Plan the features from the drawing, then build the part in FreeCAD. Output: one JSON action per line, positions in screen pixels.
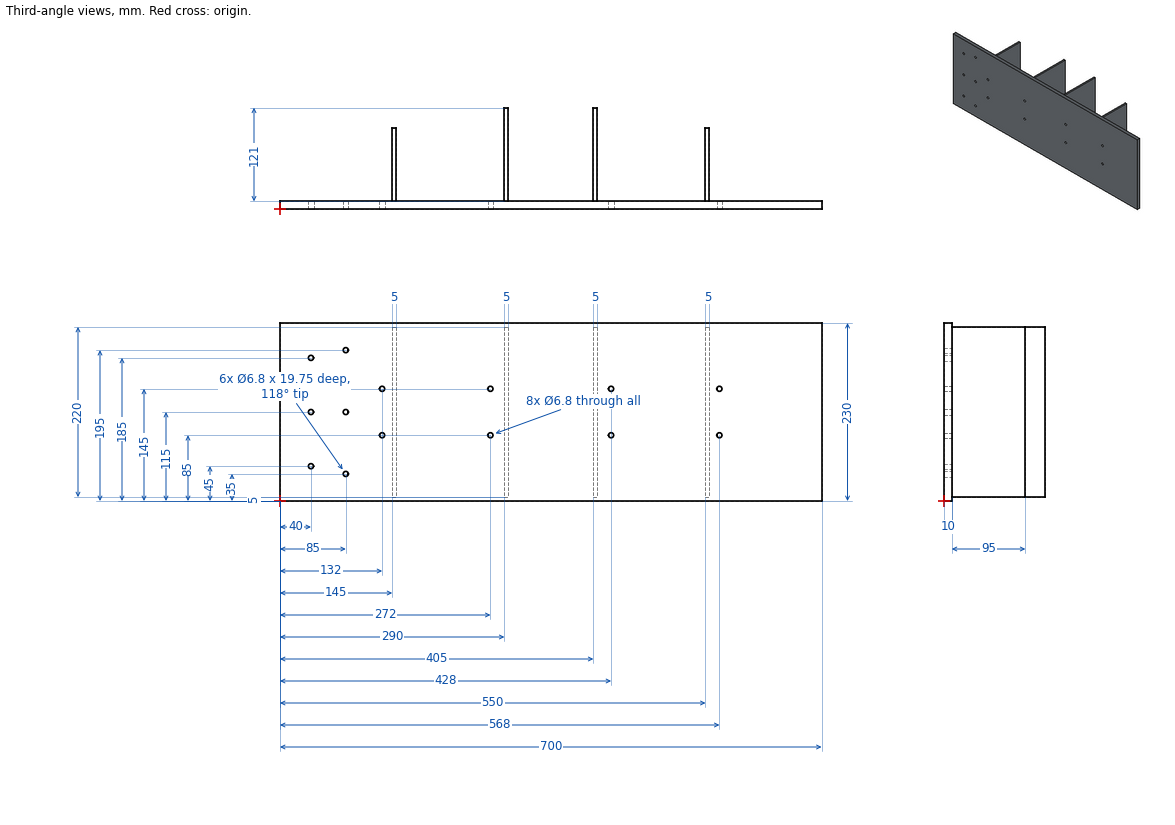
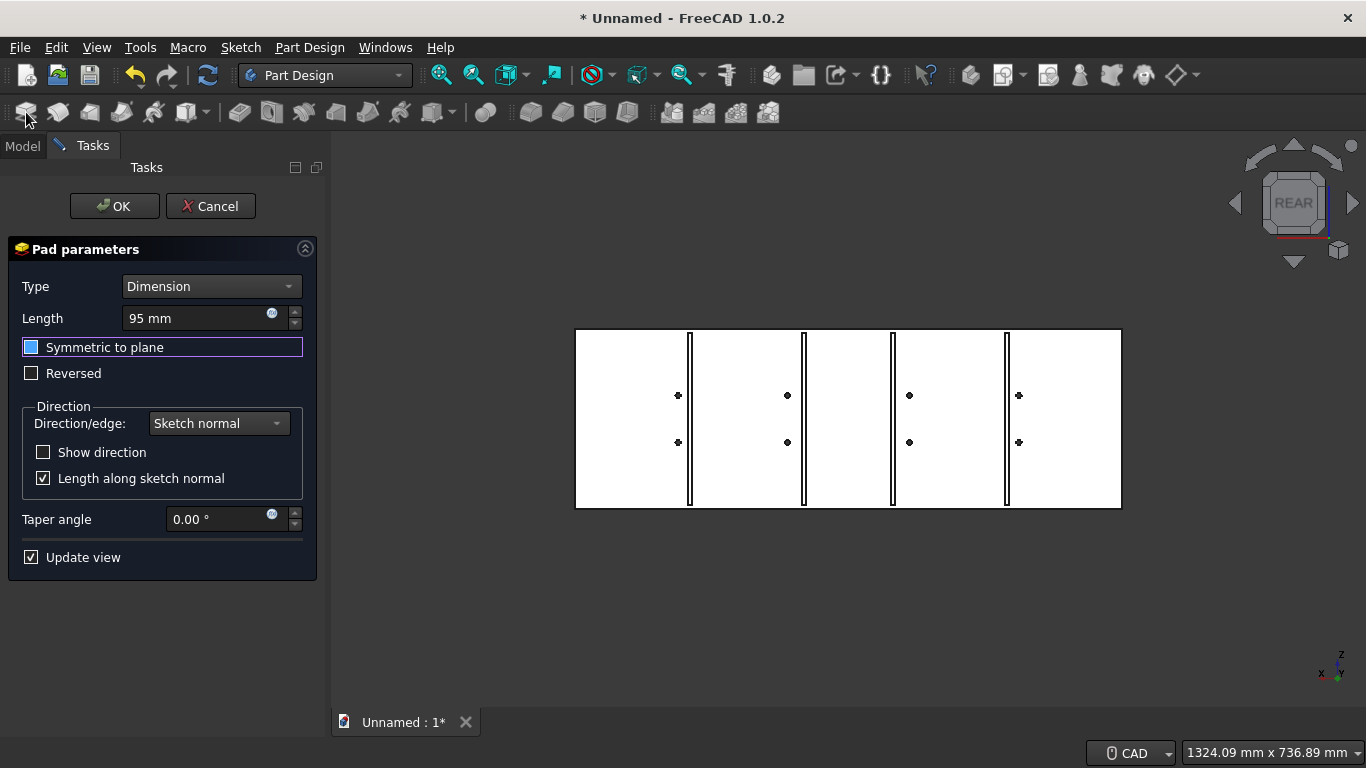
{"action": "left_click", "coordinate": [115, 206]}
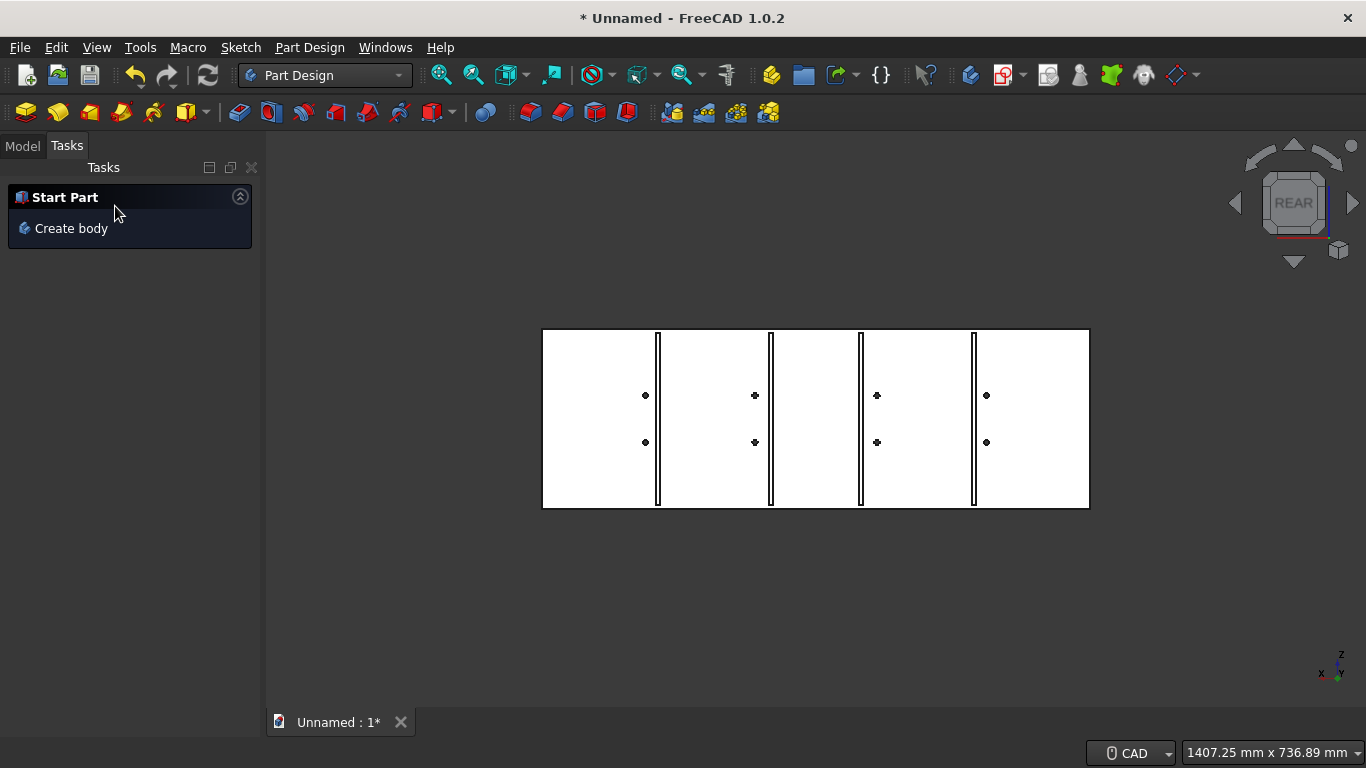
{"action": "left_click", "coordinate": [1004, 76]}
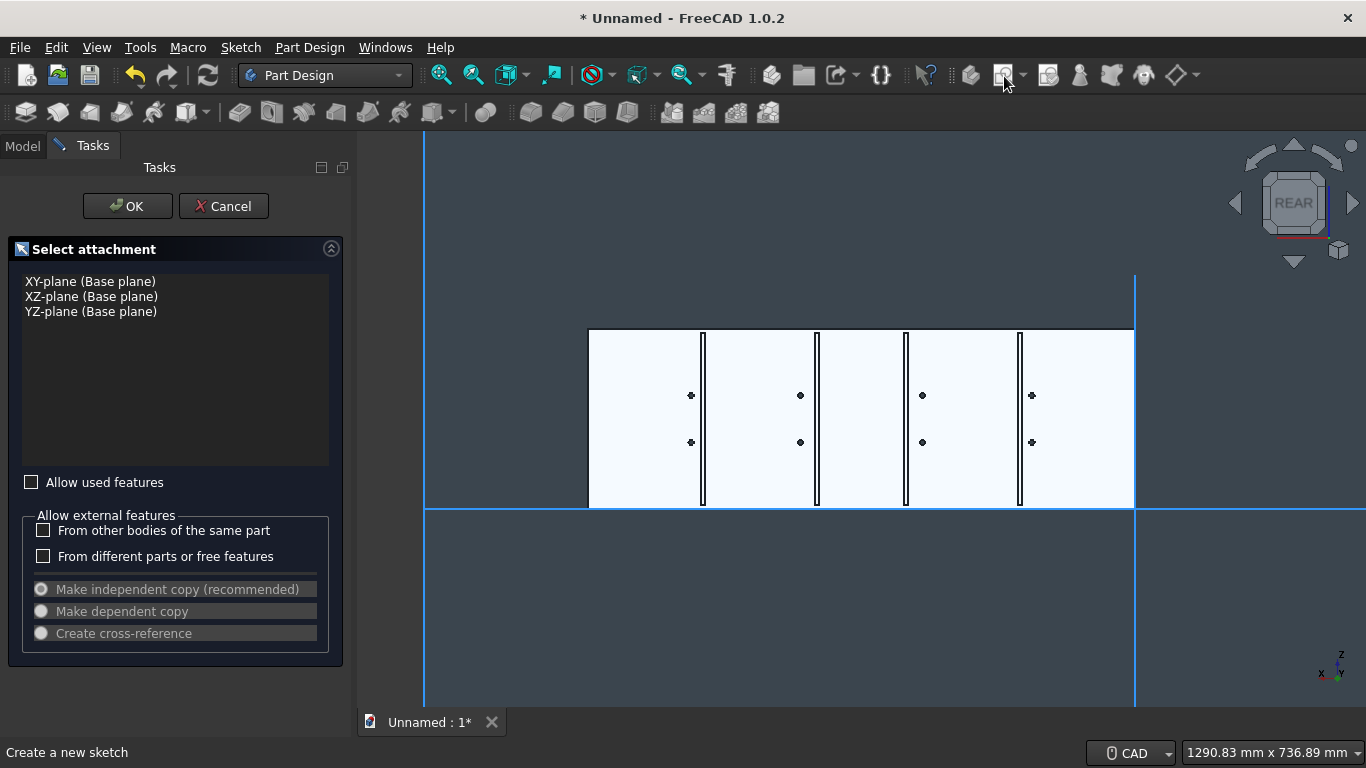
{"action": "left_click", "coordinate": [82, 296]}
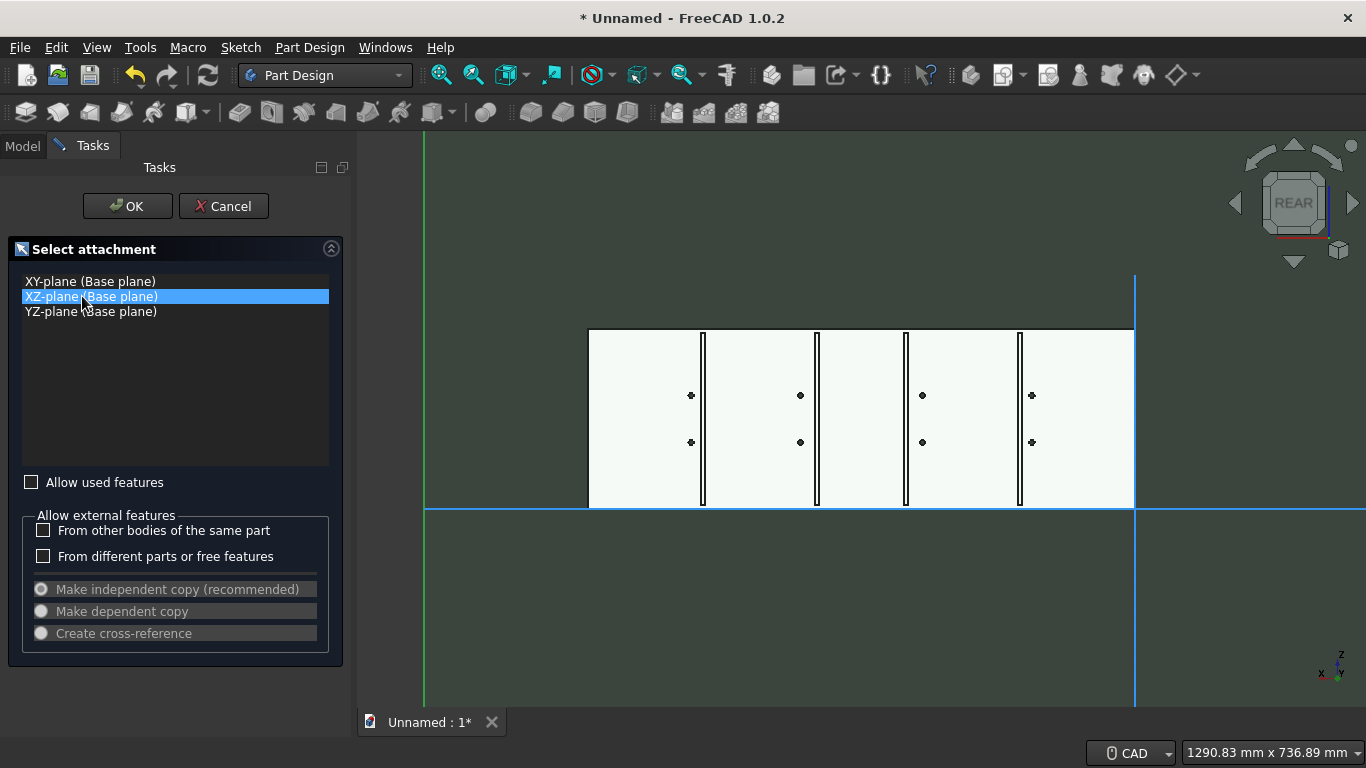
{"action": "left_click", "coordinate": [128, 206]}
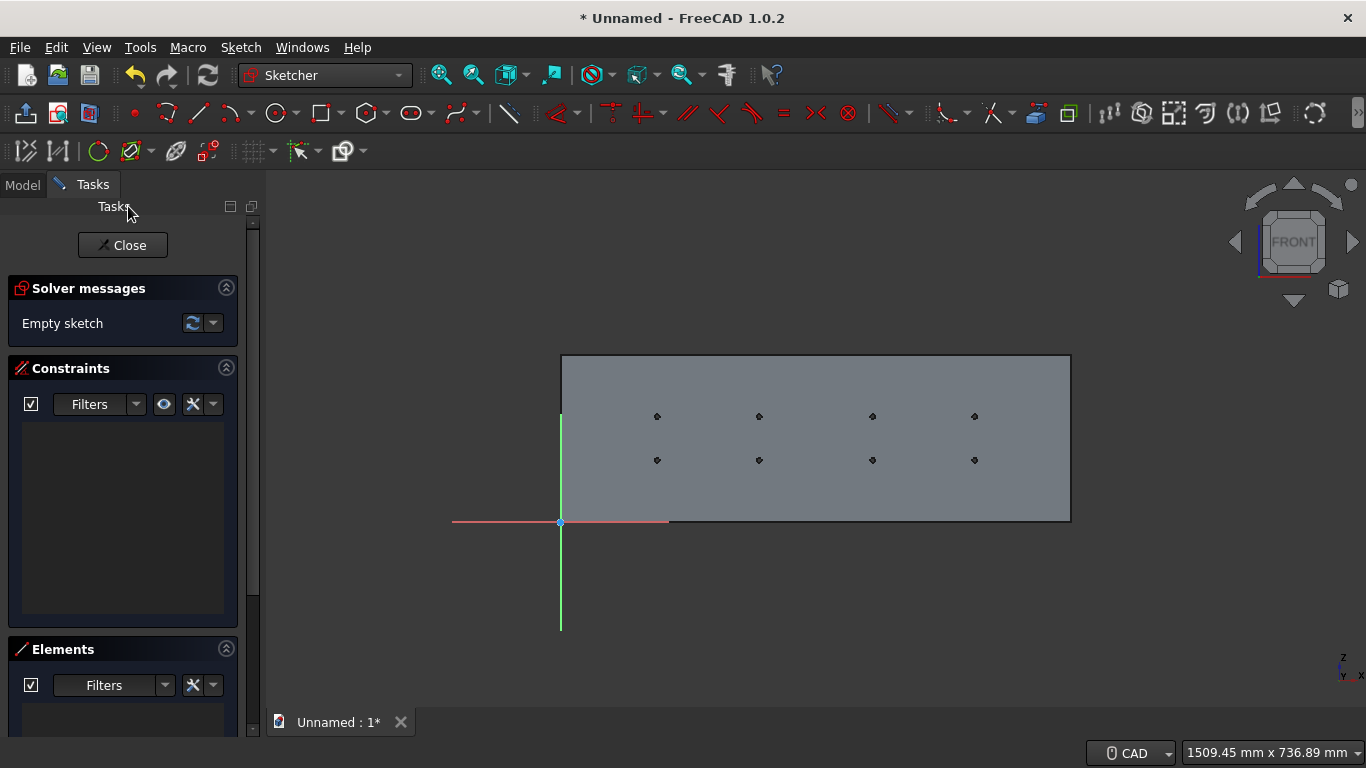
{"action": "scroll", "coordinate": [467, 459], "scroll_direction": "up", "scroll_amount": 4}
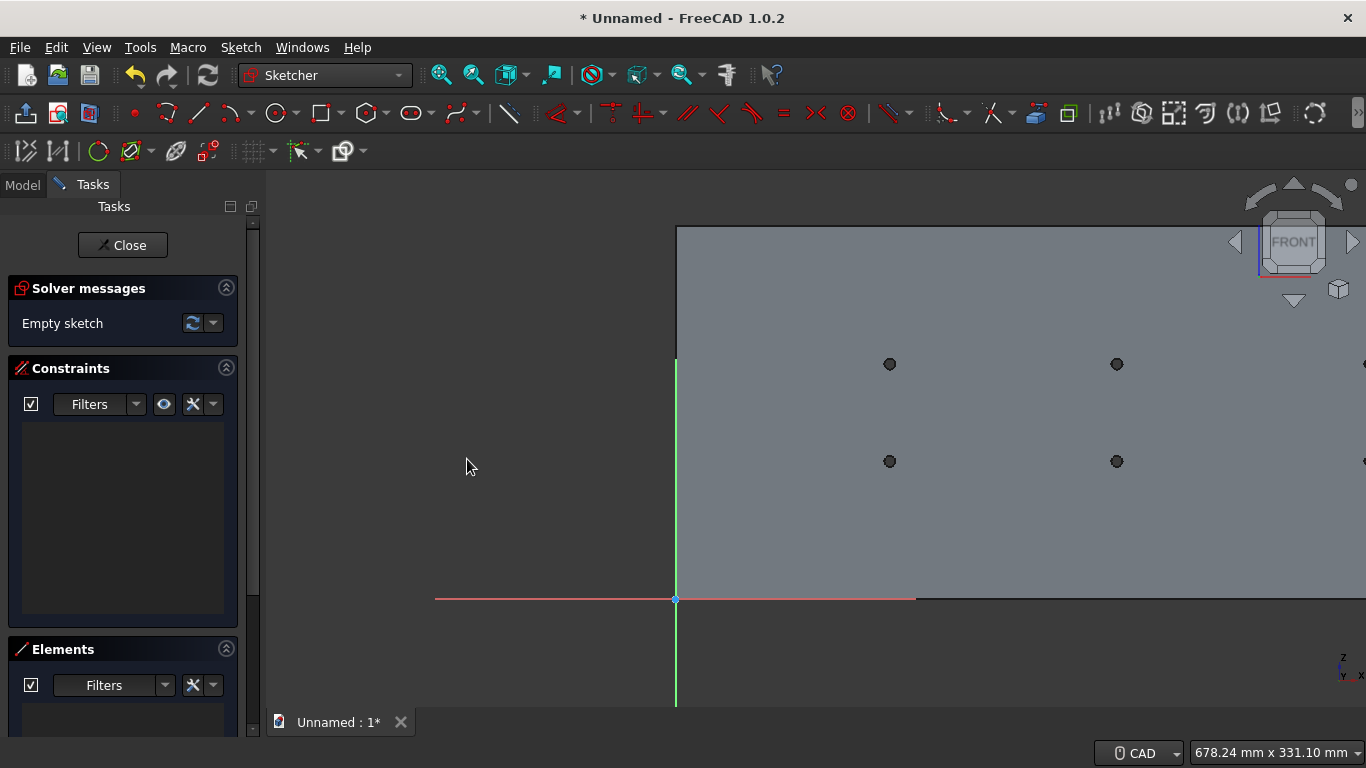
{"action": "left_click", "coordinate": [276, 114]}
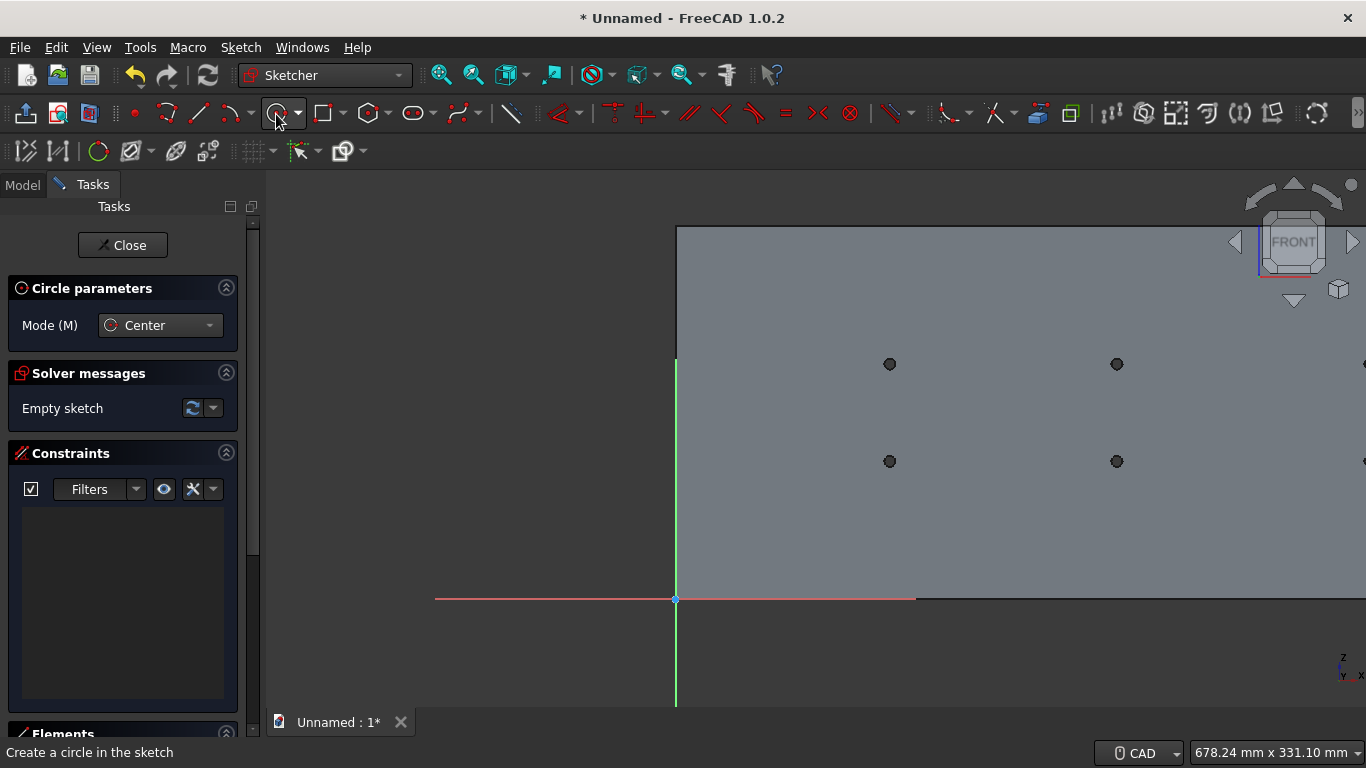
{"action": "scroll", "coordinate": [814, 542], "scroll_direction": "up", "scroll_amount": 8}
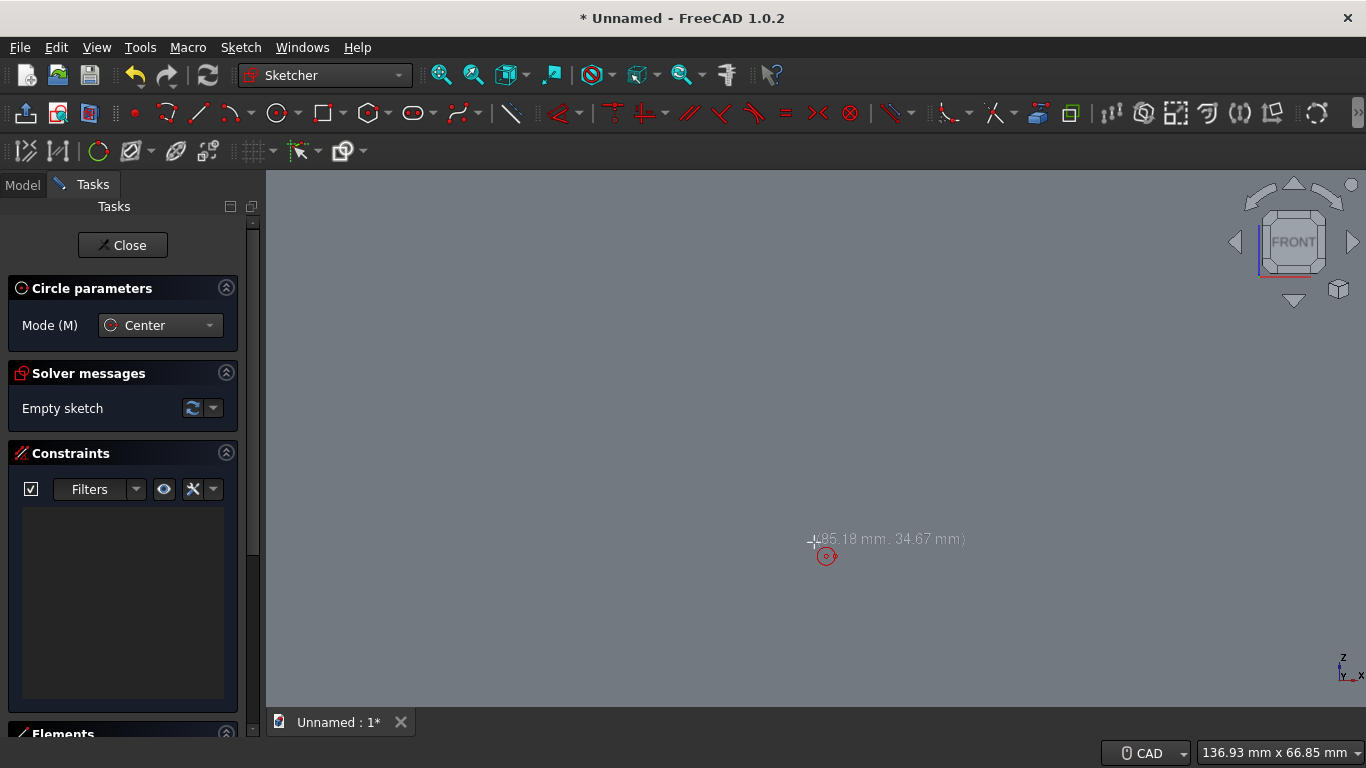
{"action": "scroll", "coordinate": [814, 543], "scroll_direction": "down", "scroll_amount": 8}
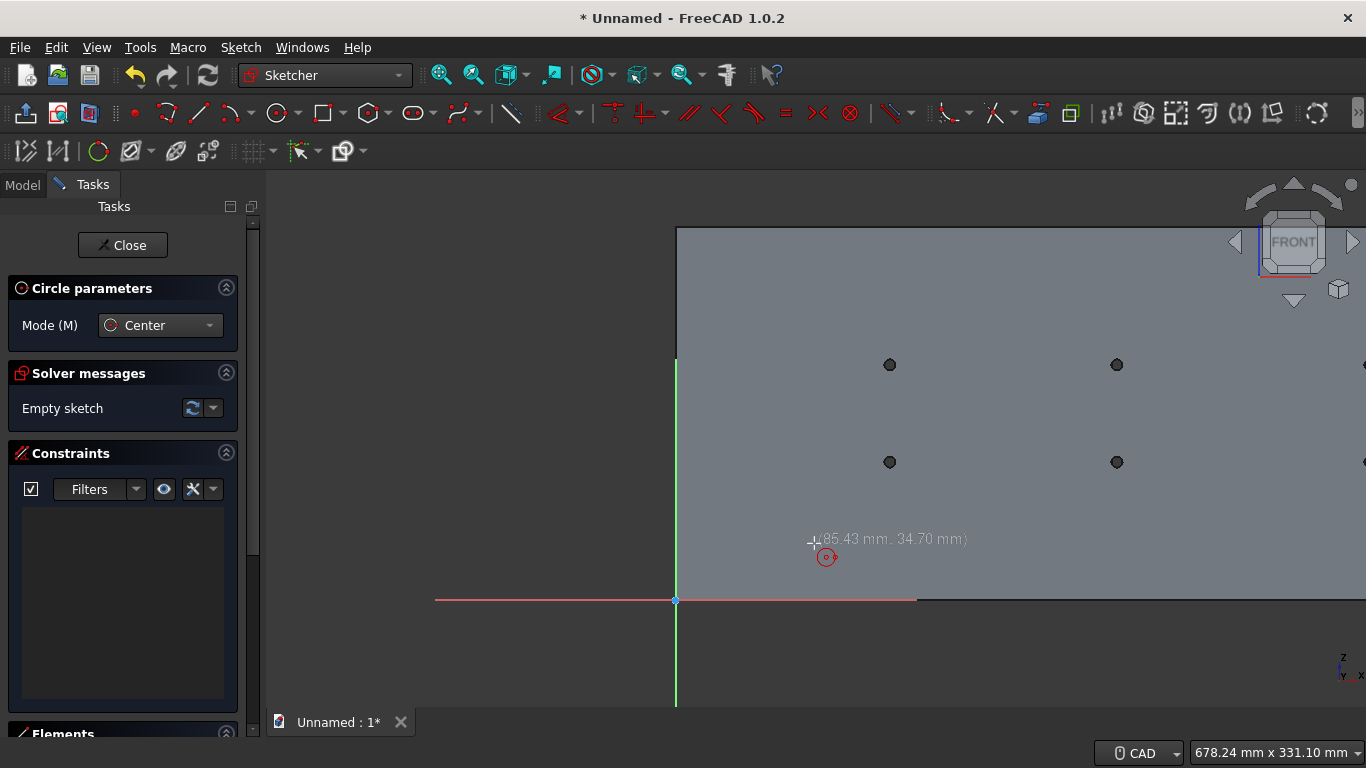
{"action": "left_click", "coordinate": [814, 543]}